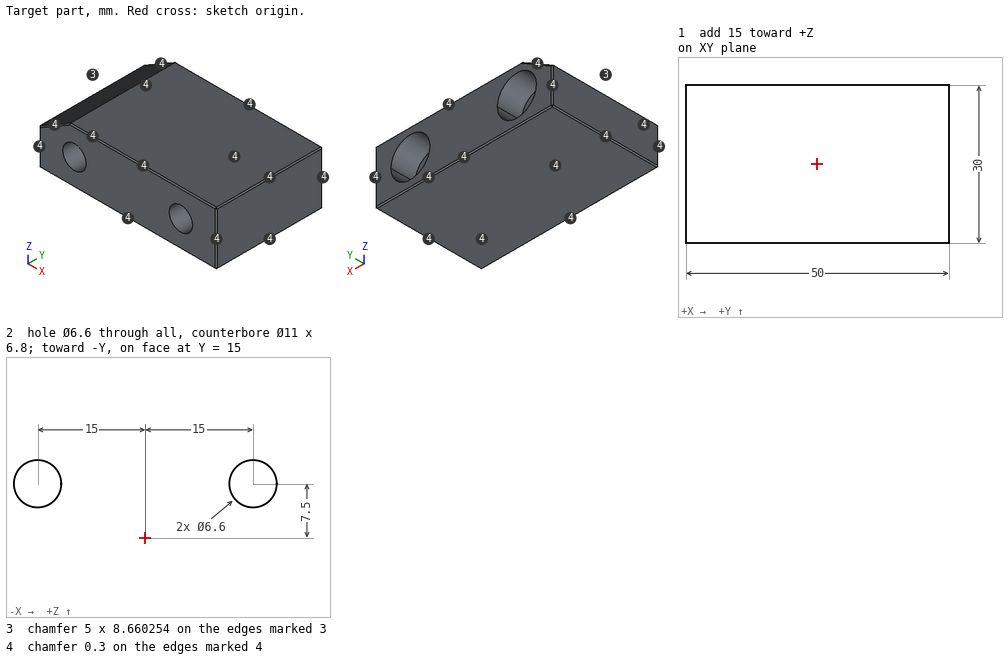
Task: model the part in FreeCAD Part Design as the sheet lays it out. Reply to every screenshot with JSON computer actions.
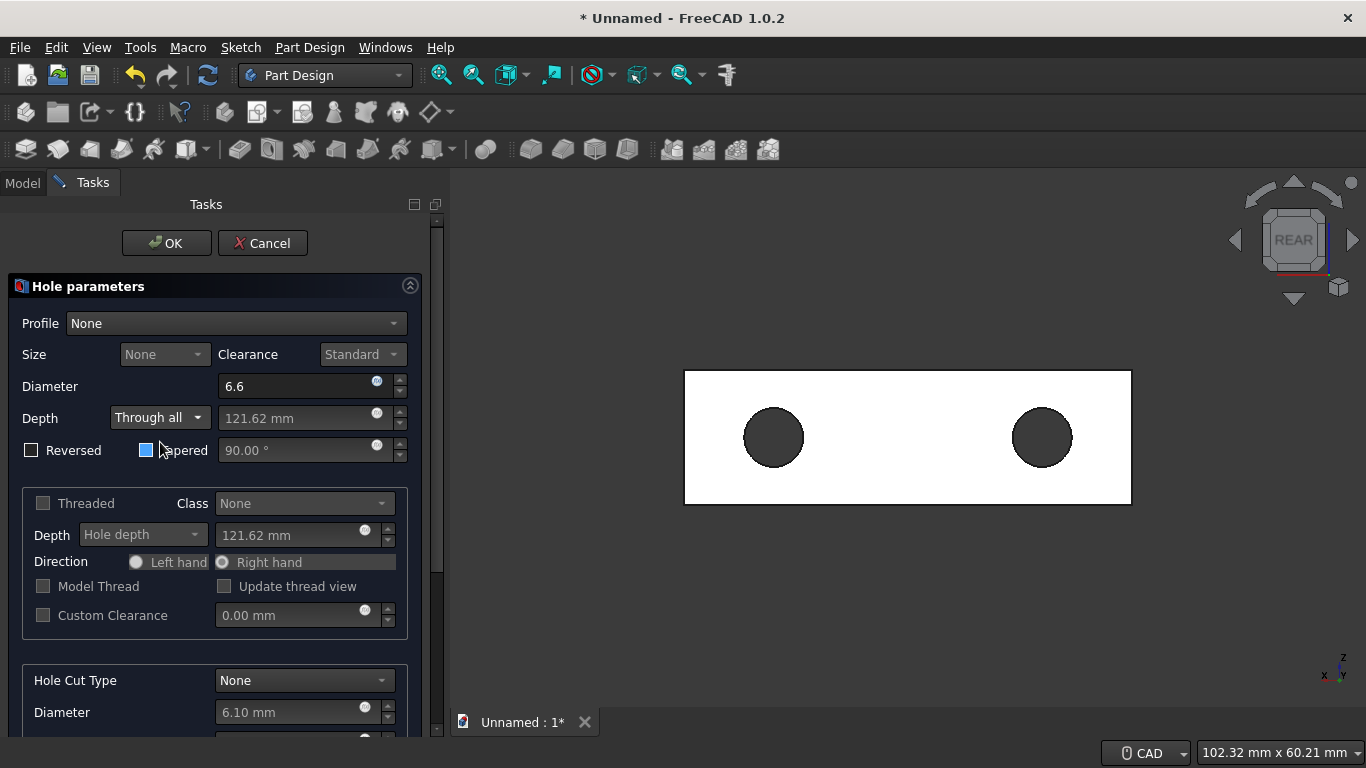
{"action": "left_click", "coordinate": [306, 680]}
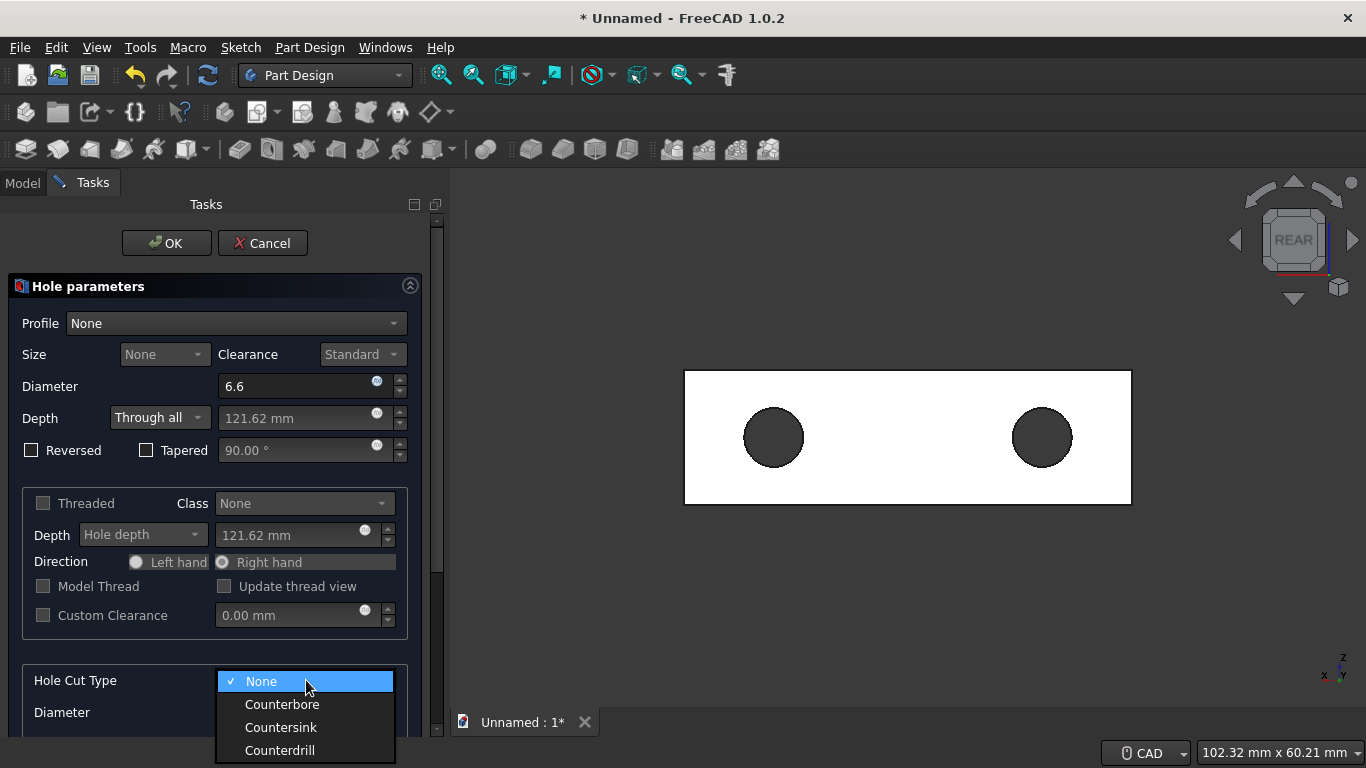
{"action": "left_click", "coordinate": [304, 704]}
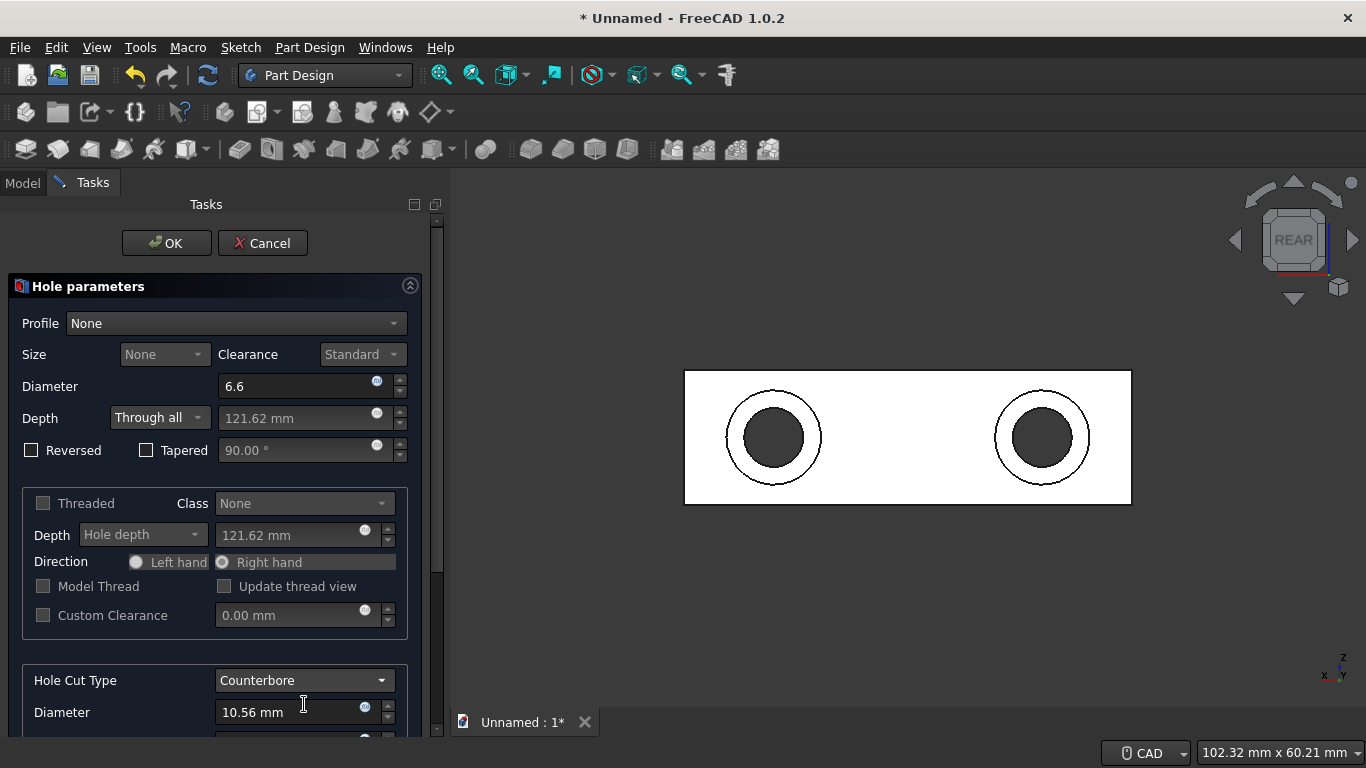
{"action": "triple_click", "coordinate": [298, 712]}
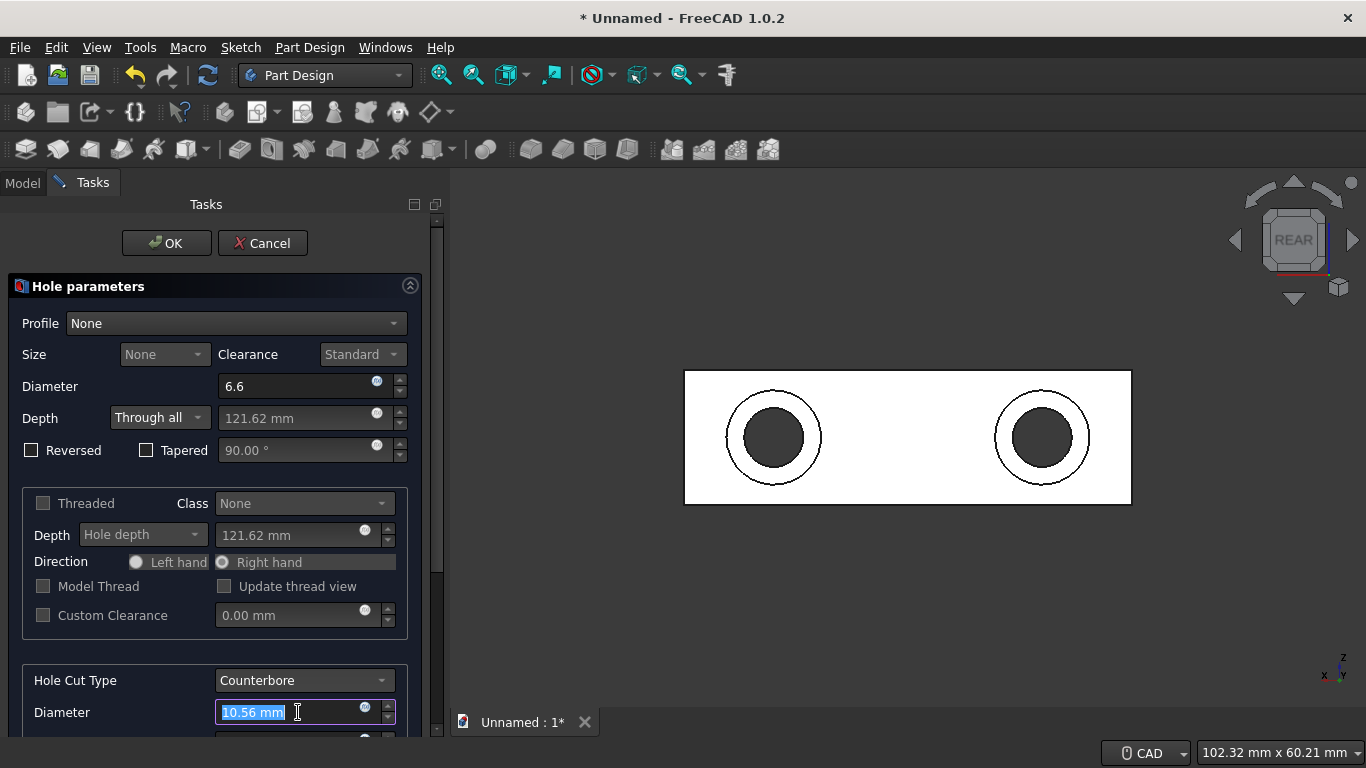
{"action": "type", "text": "11"}
{"action": "key", "text": "Tab"}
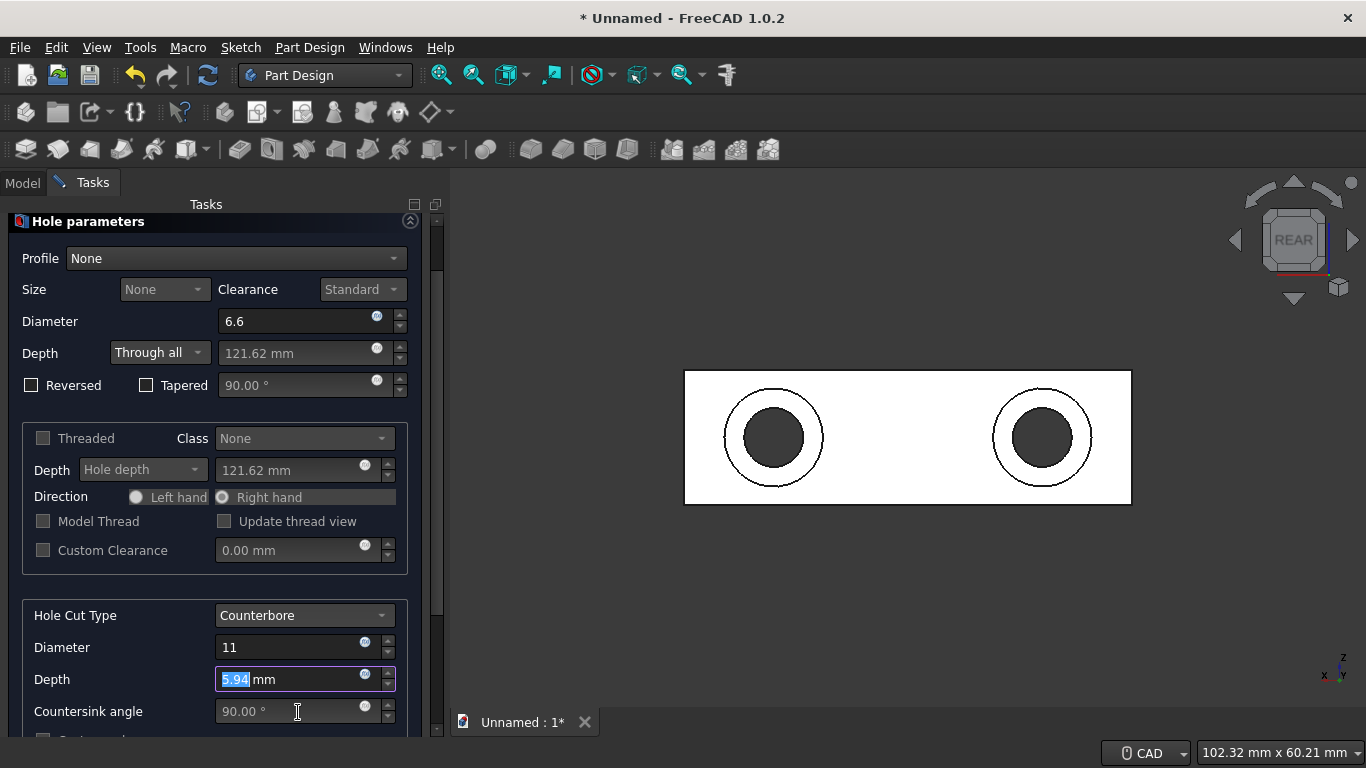
{"action": "type", "text": "6.8"}
{"action": "key", "text": "Tab"}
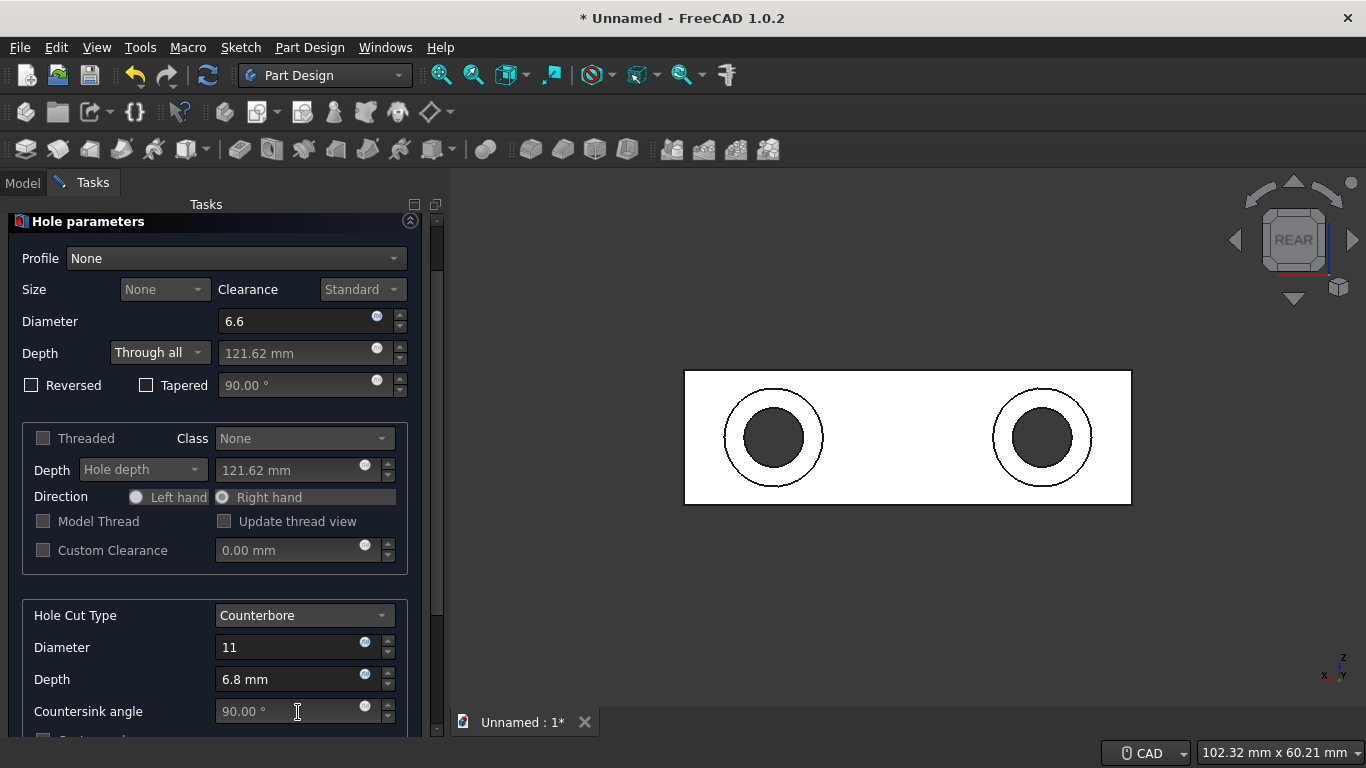
{"action": "scroll", "coordinate": [437, 475], "scroll_direction": "up", "scroll_amount": 2}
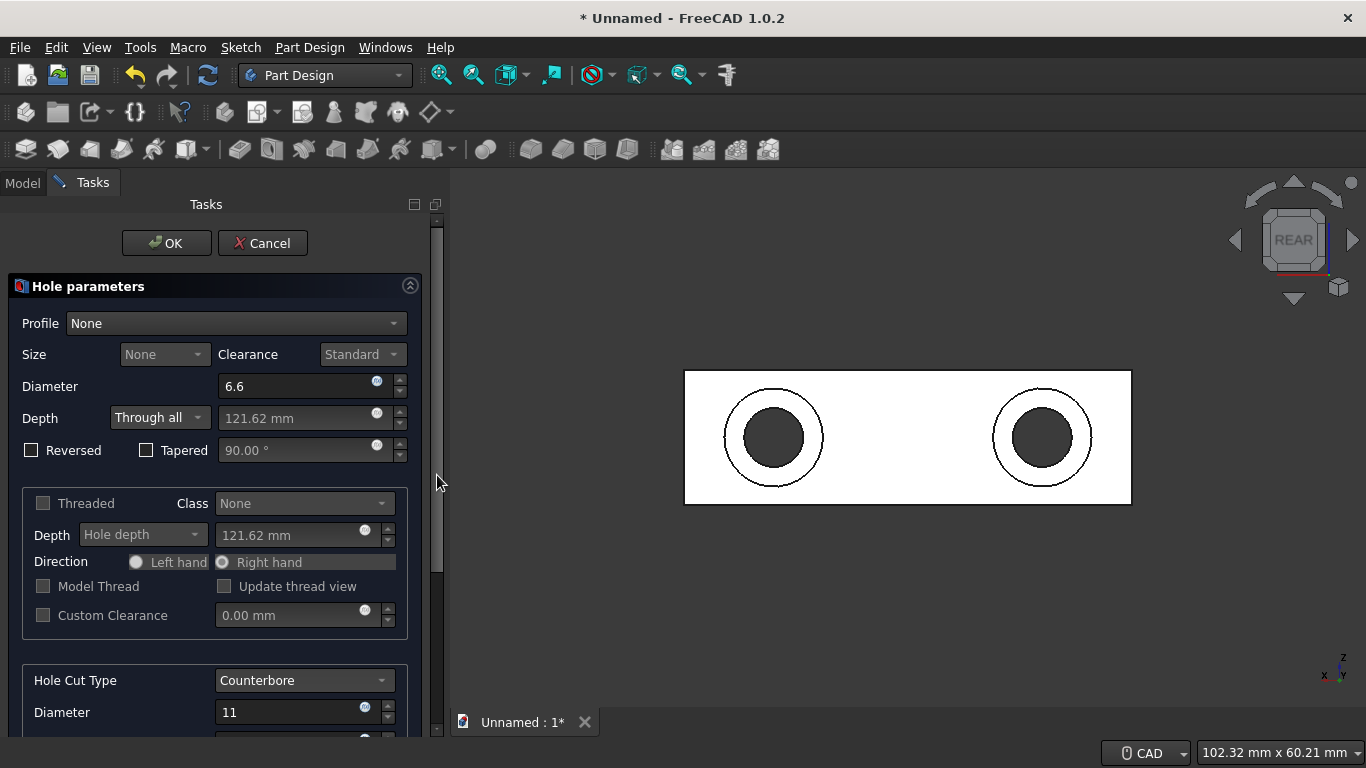
{"action": "left_click", "coordinate": [167, 243]}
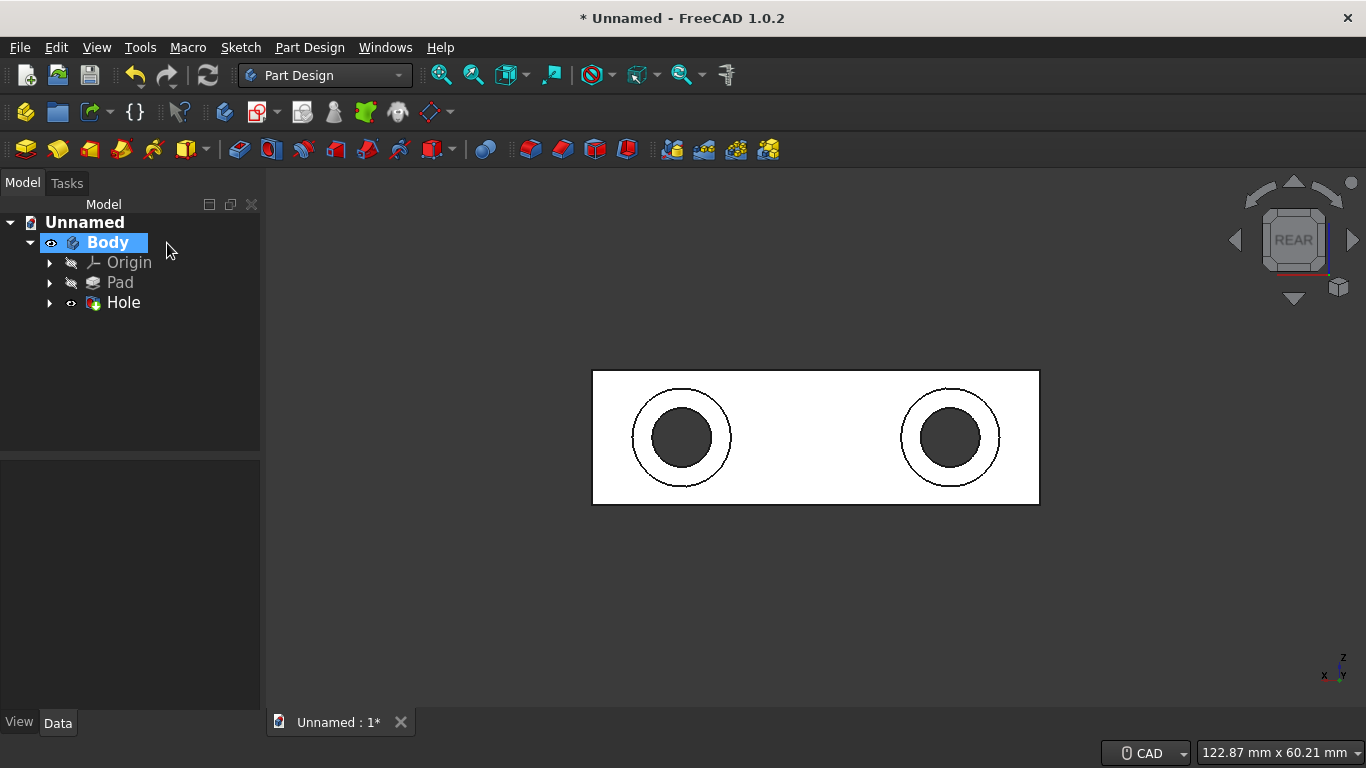
{"action": "left_click", "coordinate": [442, 76]}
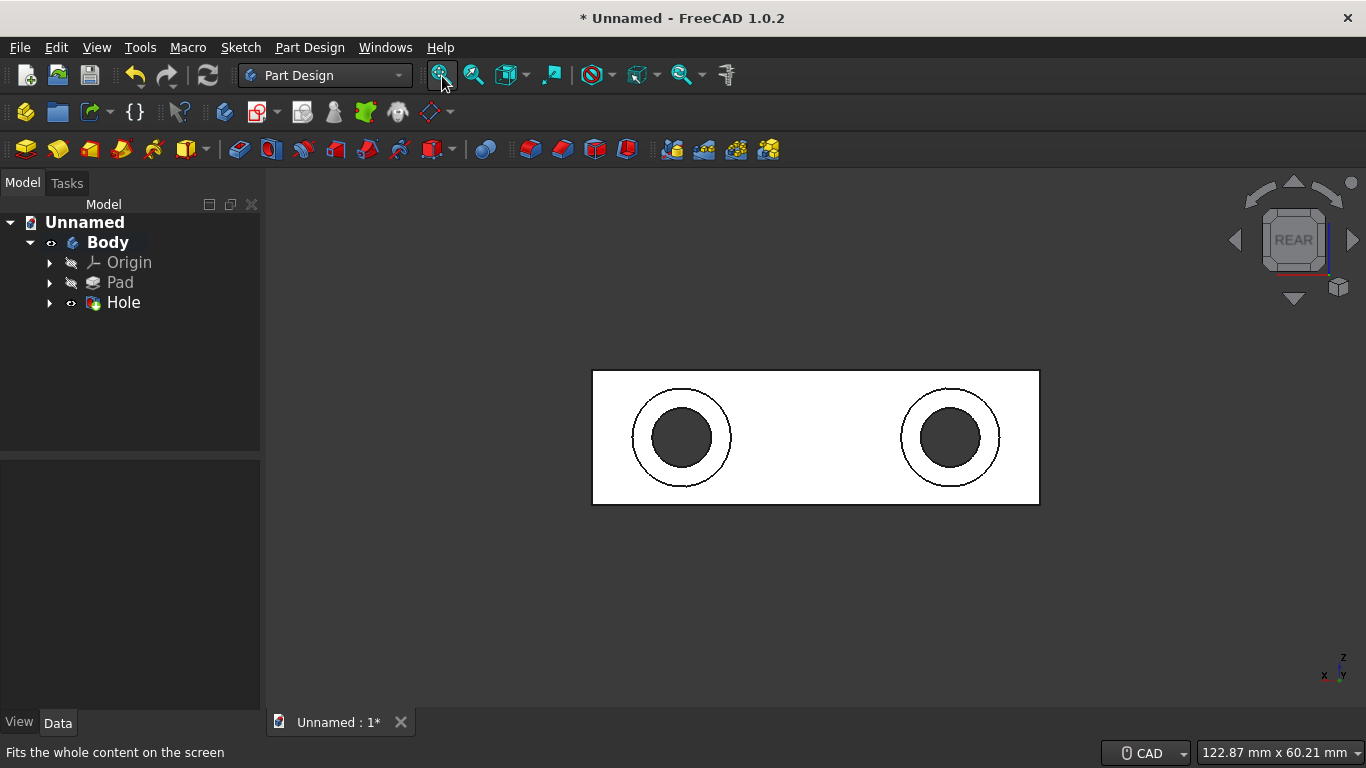
{"action": "key", "text": "0"}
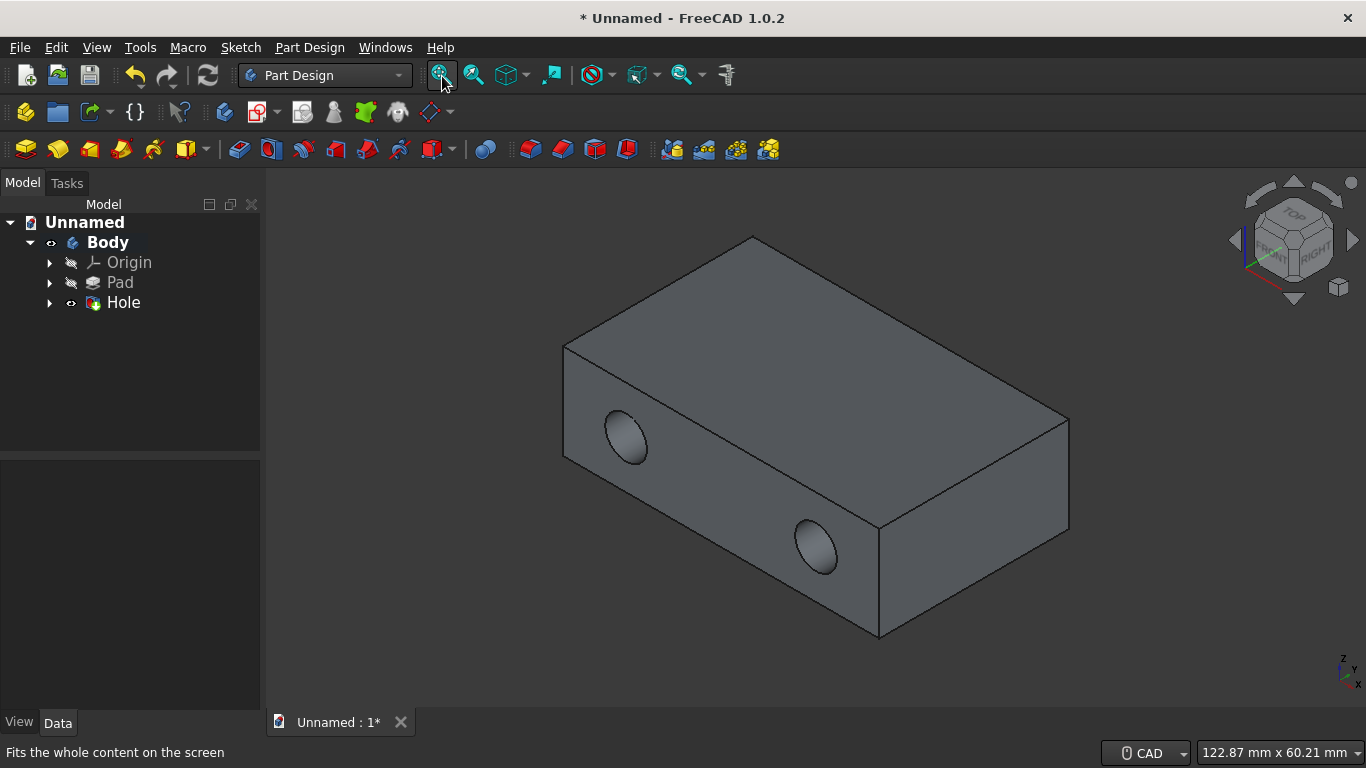
{"action": "key", "text": "2"}